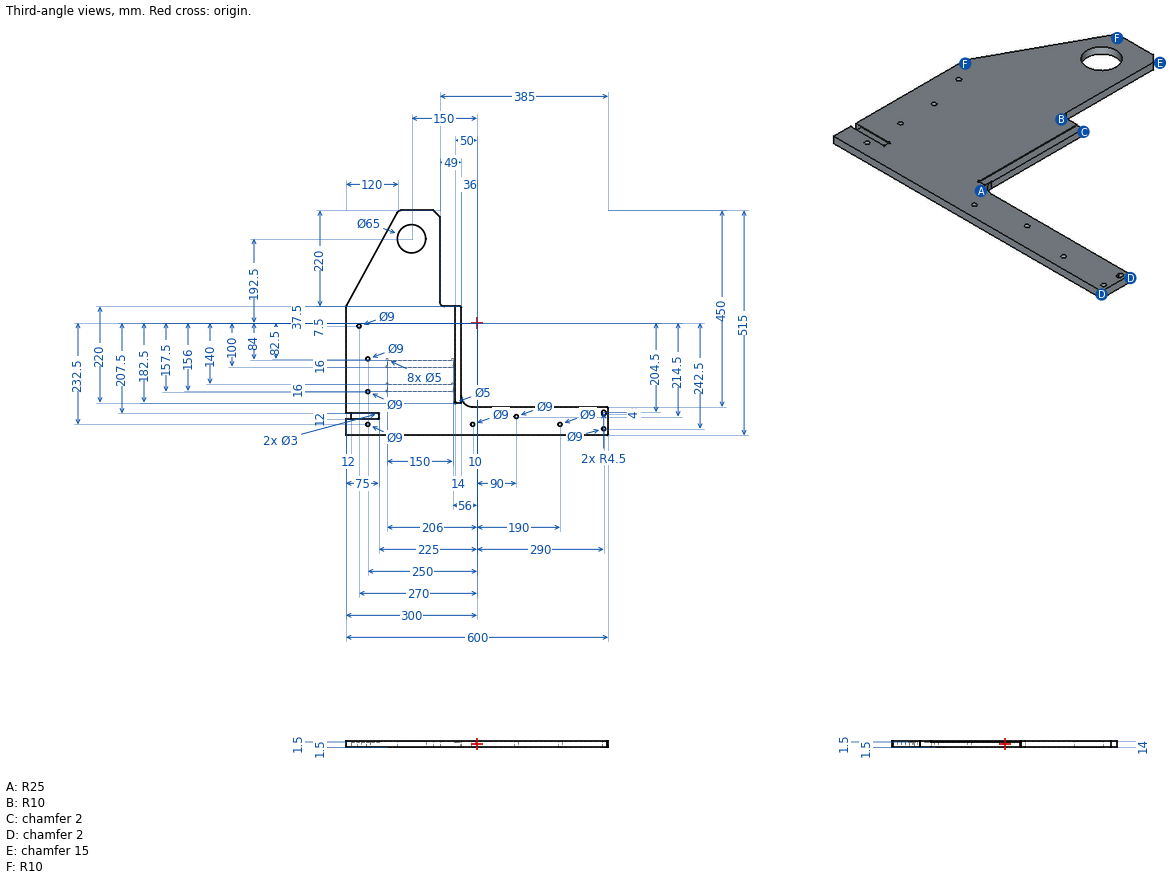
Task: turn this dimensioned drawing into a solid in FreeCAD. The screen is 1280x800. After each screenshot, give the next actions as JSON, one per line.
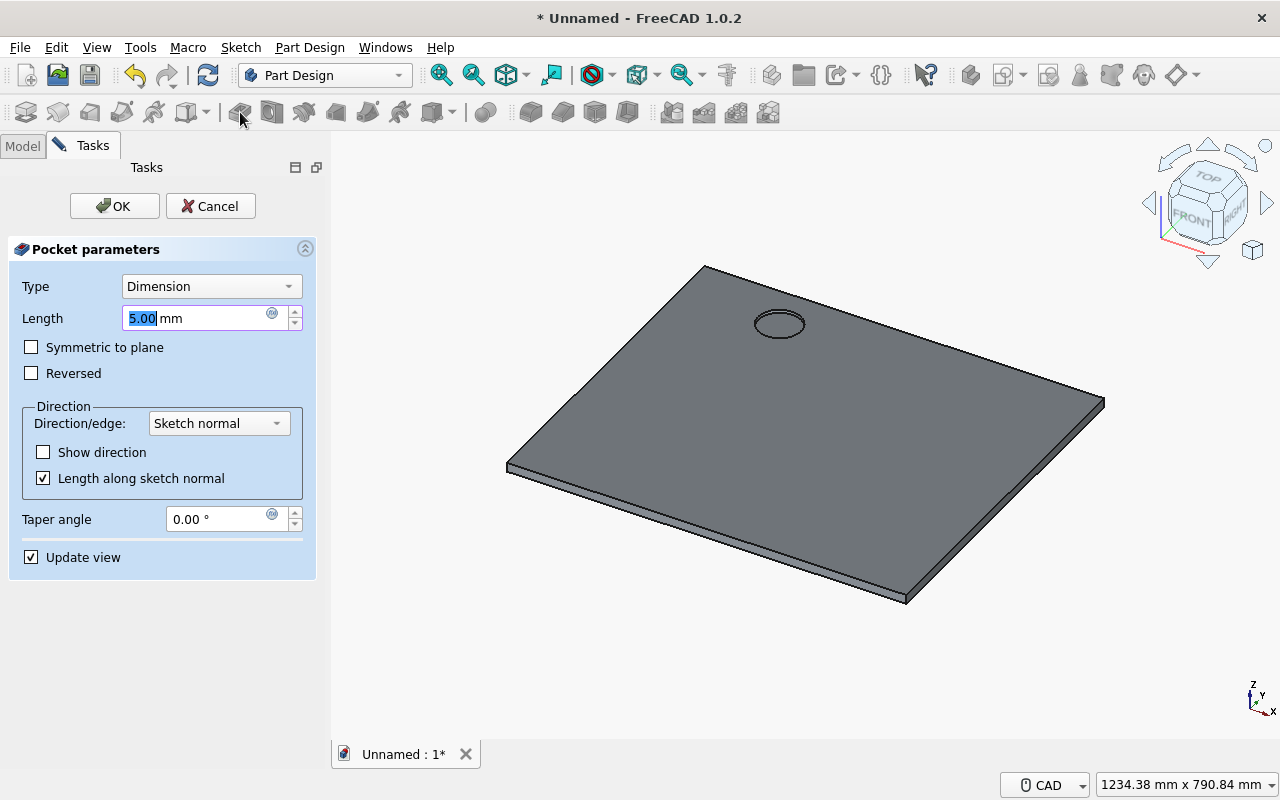
{"action": "left_click", "coordinate": [212, 286]}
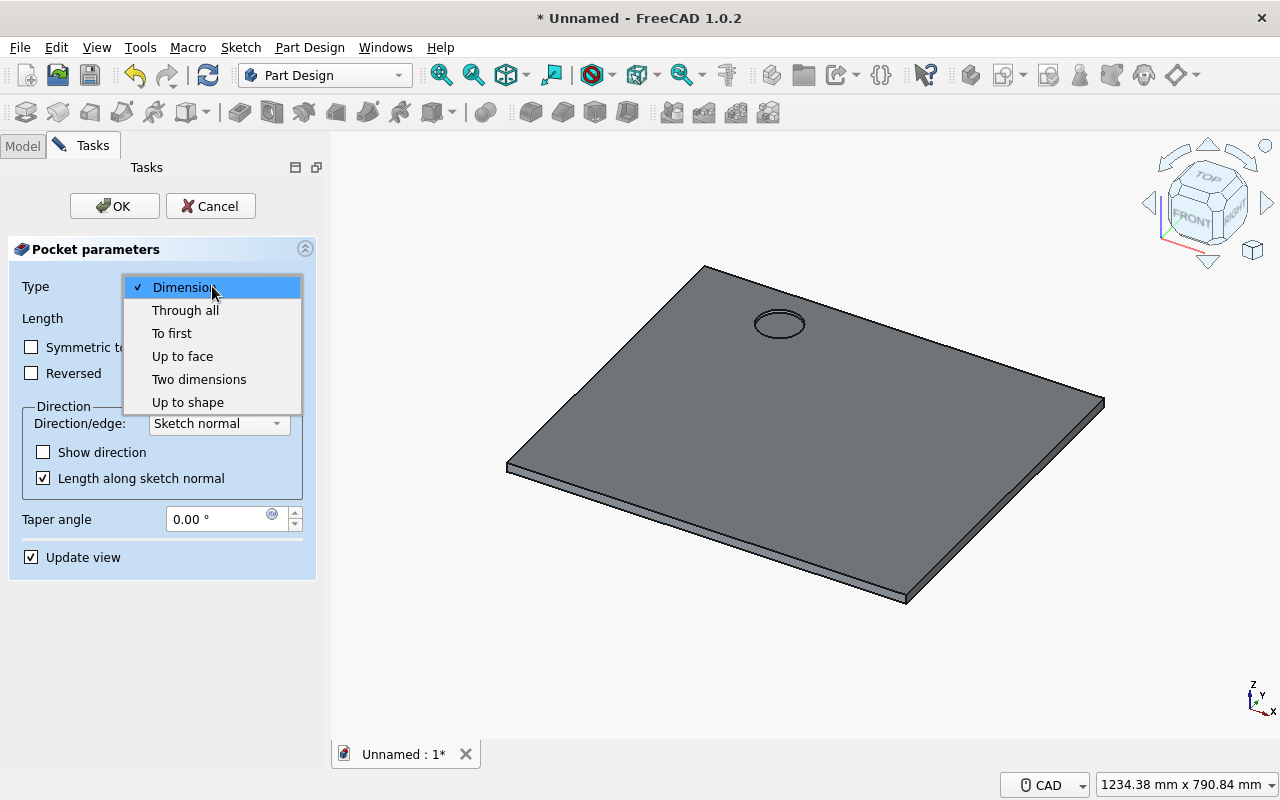
{"action": "left_click", "coordinate": [212, 334]}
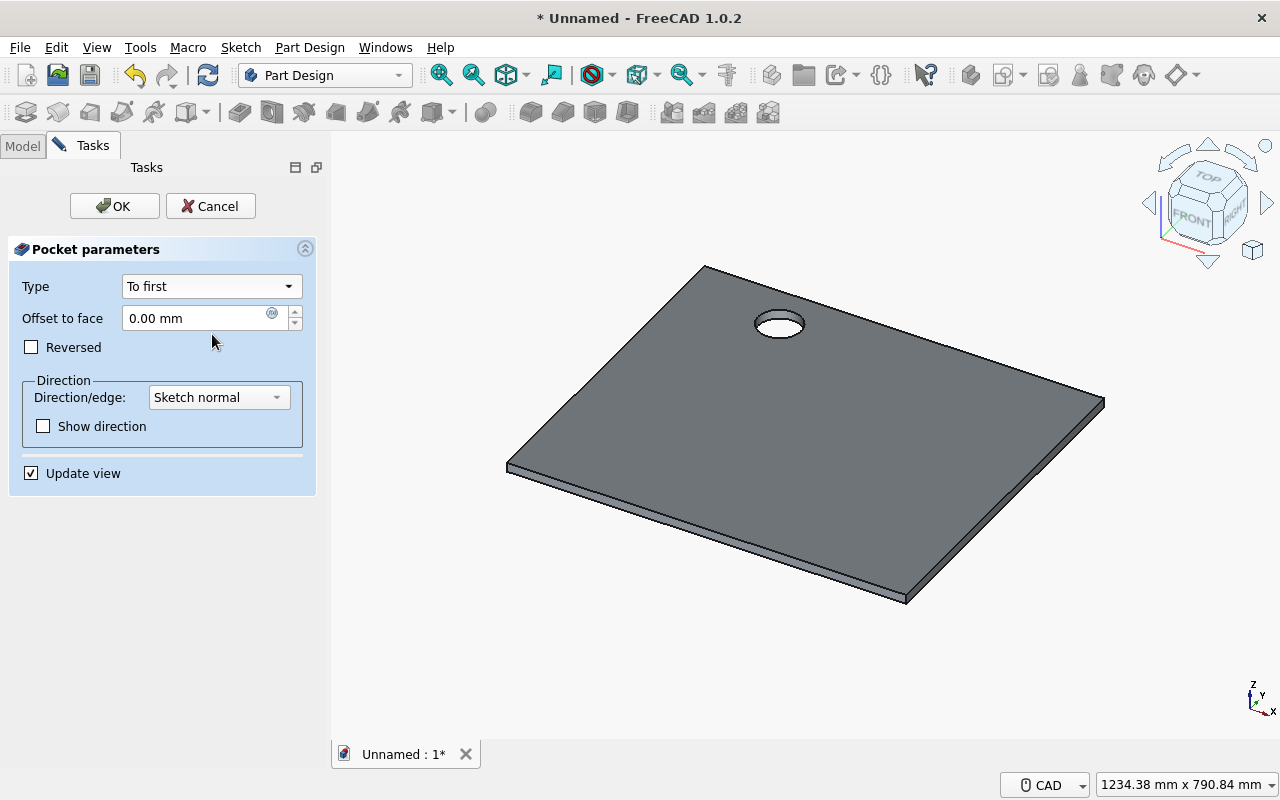
{"action": "left_click", "coordinate": [115, 206]}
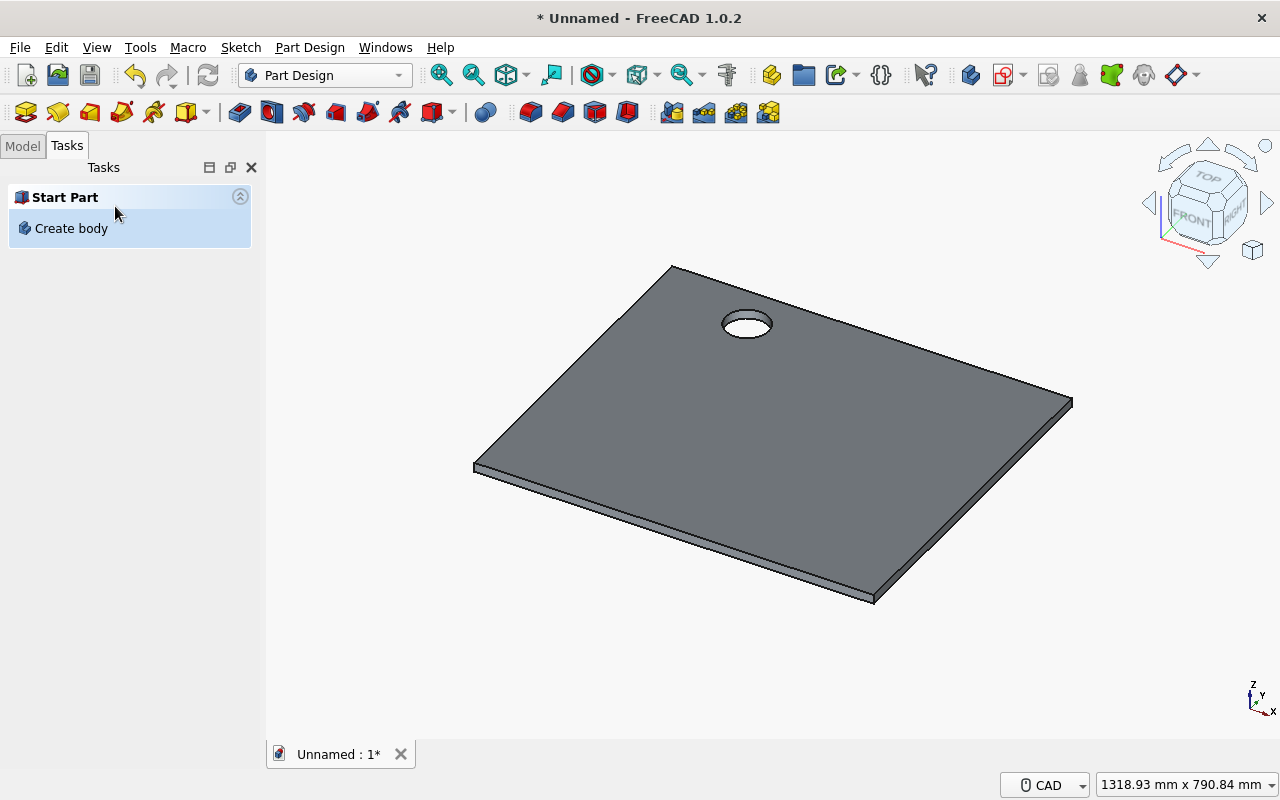
{"action": "key", "text": "5"}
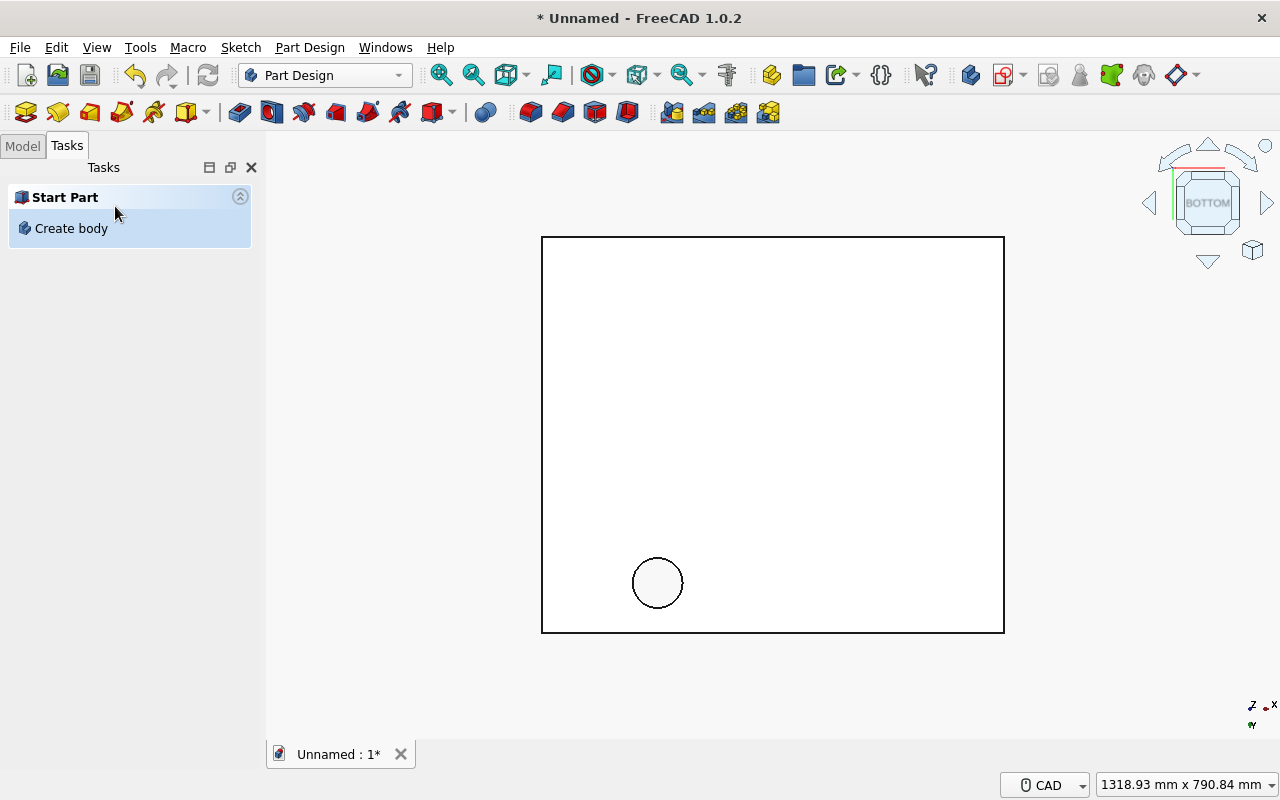
{"action": "left_click", "coordinate": [839, 434]}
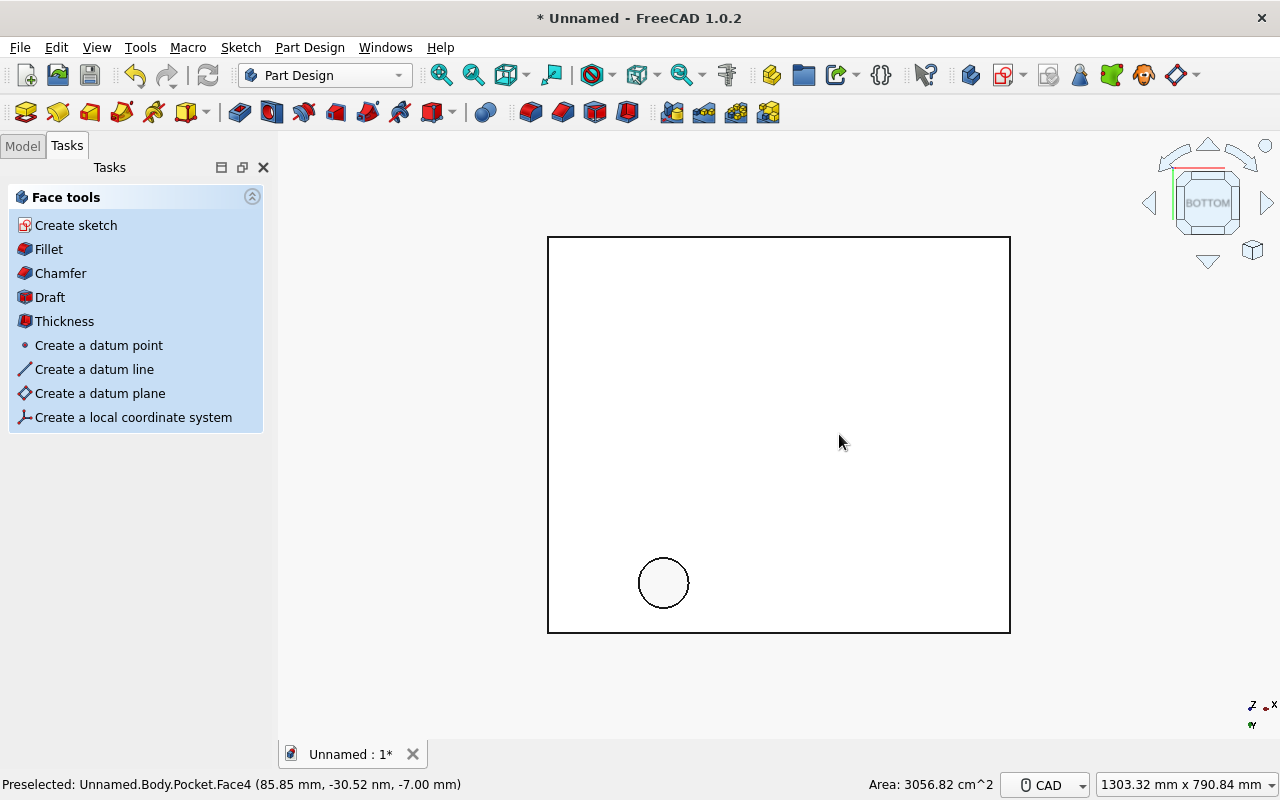
{"action": "left_click", "coordinate": [1004, 76]}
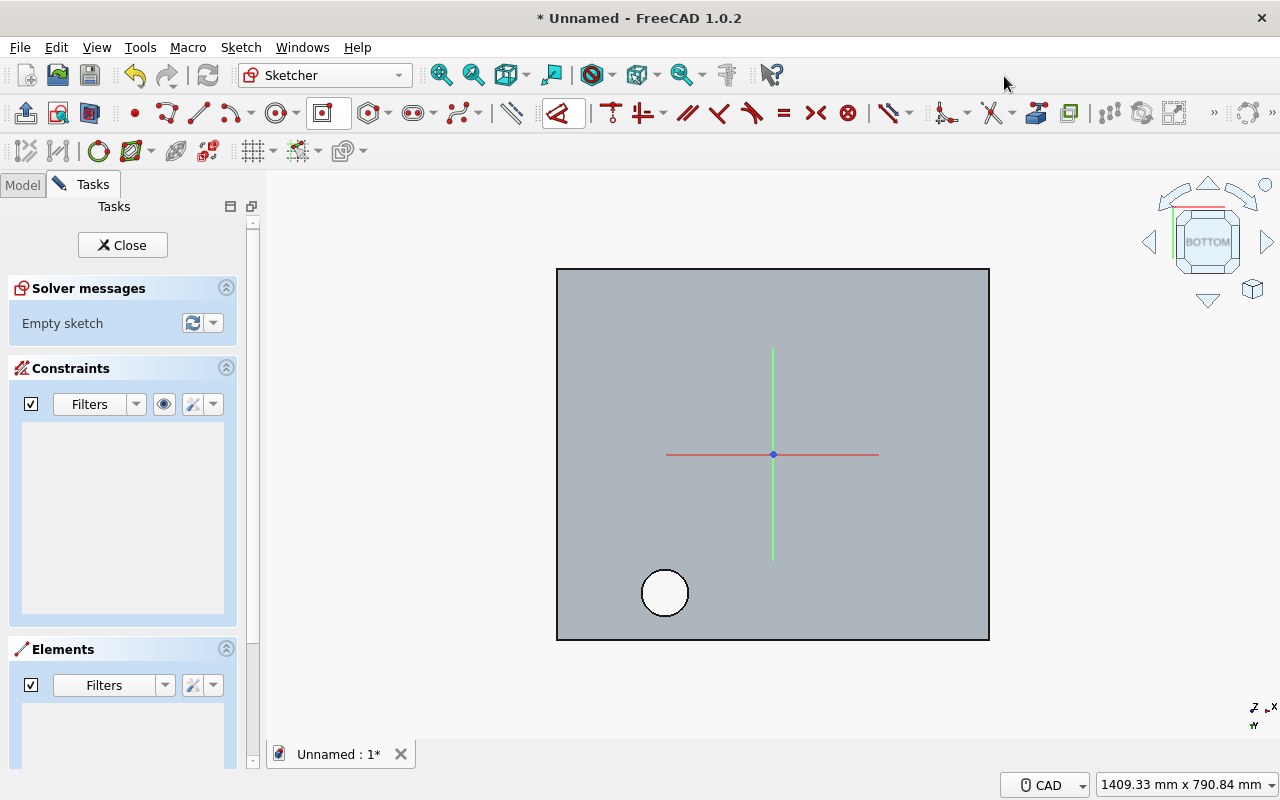
{"action": "scroll", "coordinate": [572, 449], "scroll_direction": "up", "scroll_amount": 15}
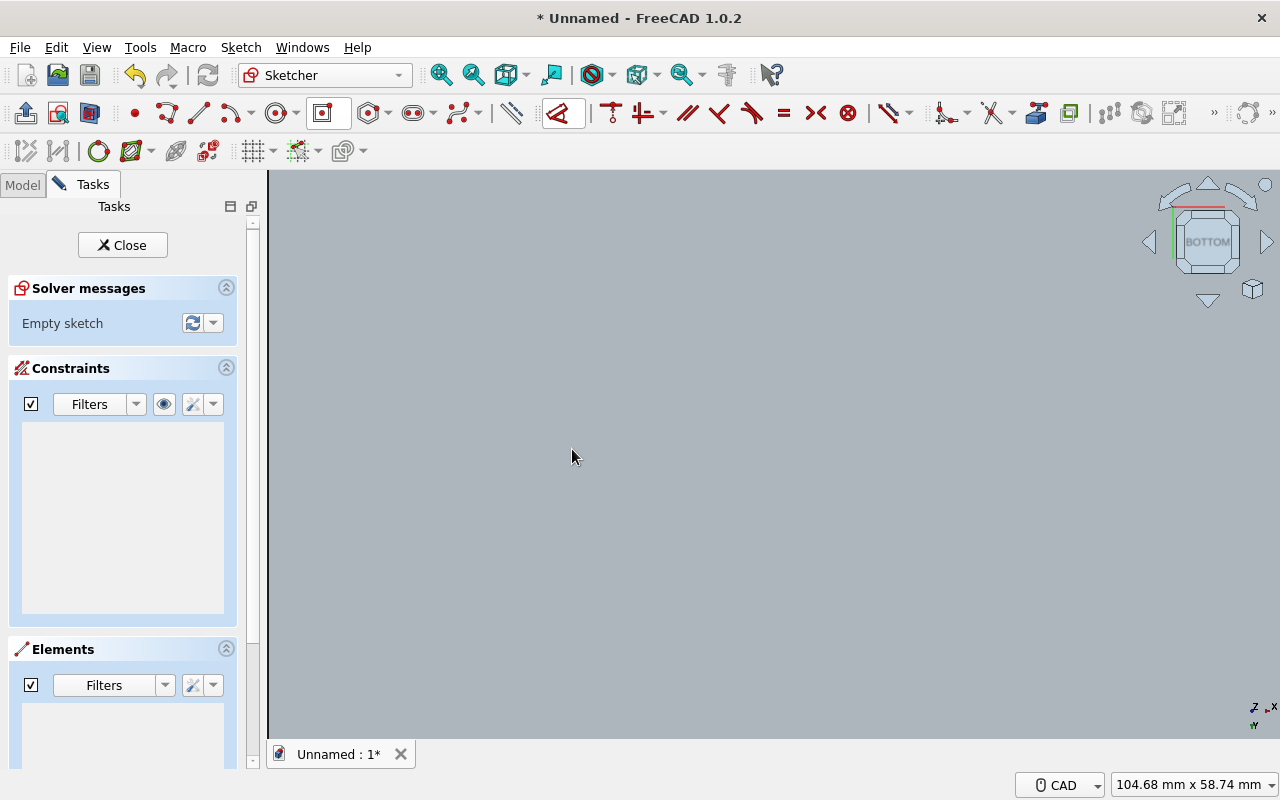
{"action": "scroll", "coordinate": [700, 434], "scroll_direction": "up", "scroll_amount": 5}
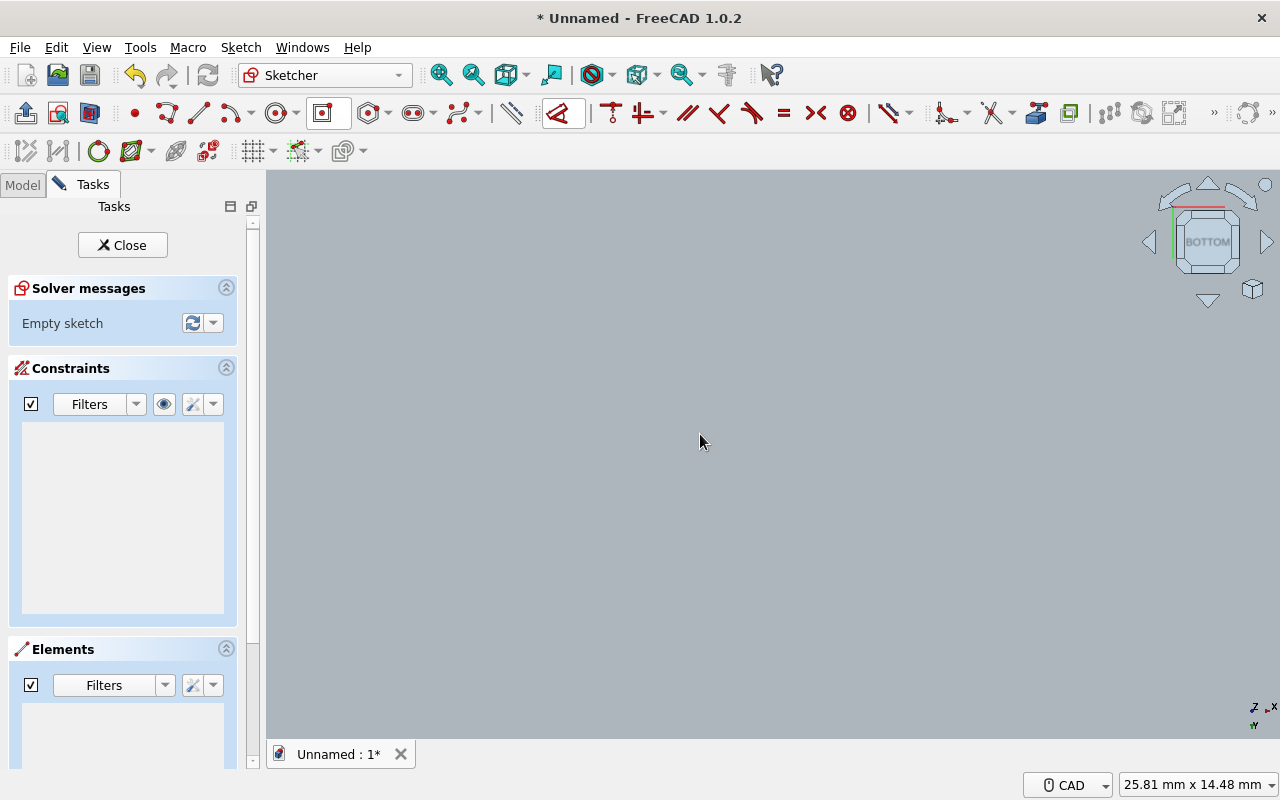
{"action": "left_click", "coordinate": [276, 114]}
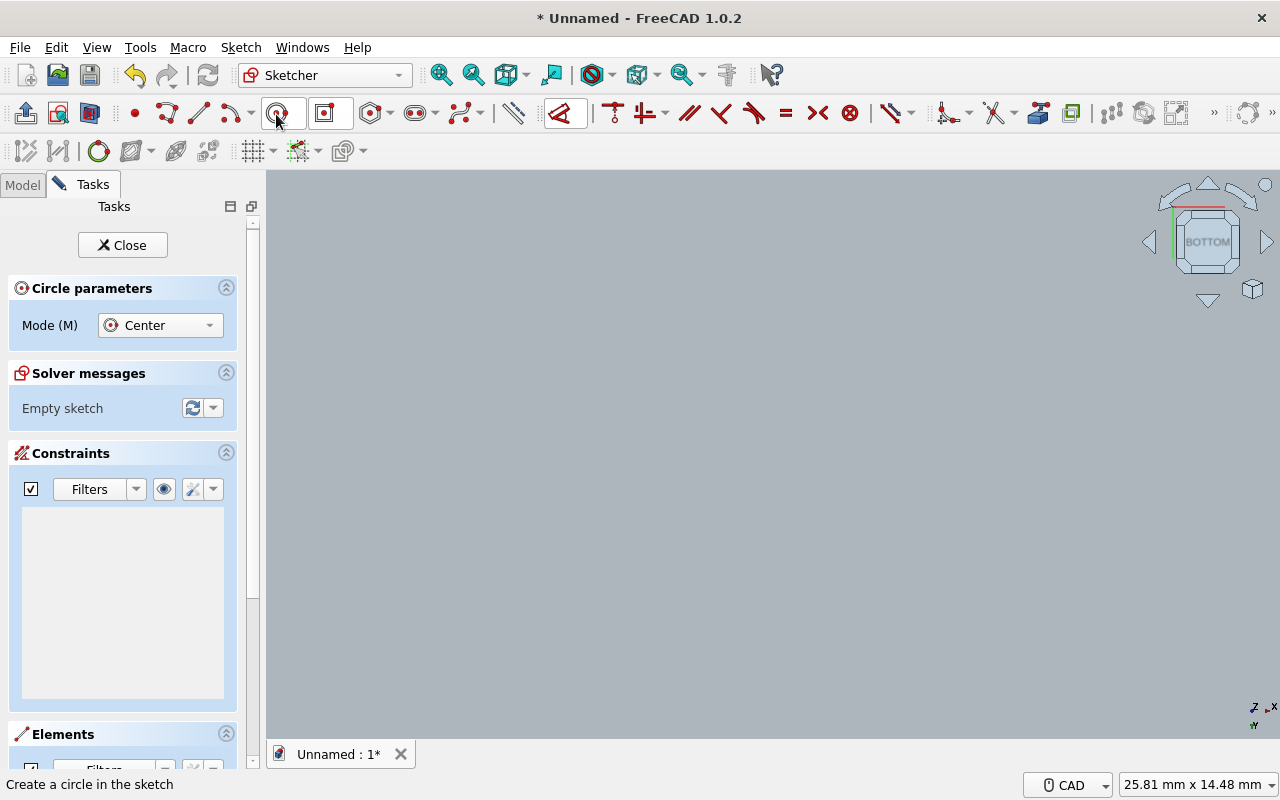
{"action": "left_click", "coordinate": [703, 454]}
{"action": "mouse_move", "coordinate": [828, 329]}